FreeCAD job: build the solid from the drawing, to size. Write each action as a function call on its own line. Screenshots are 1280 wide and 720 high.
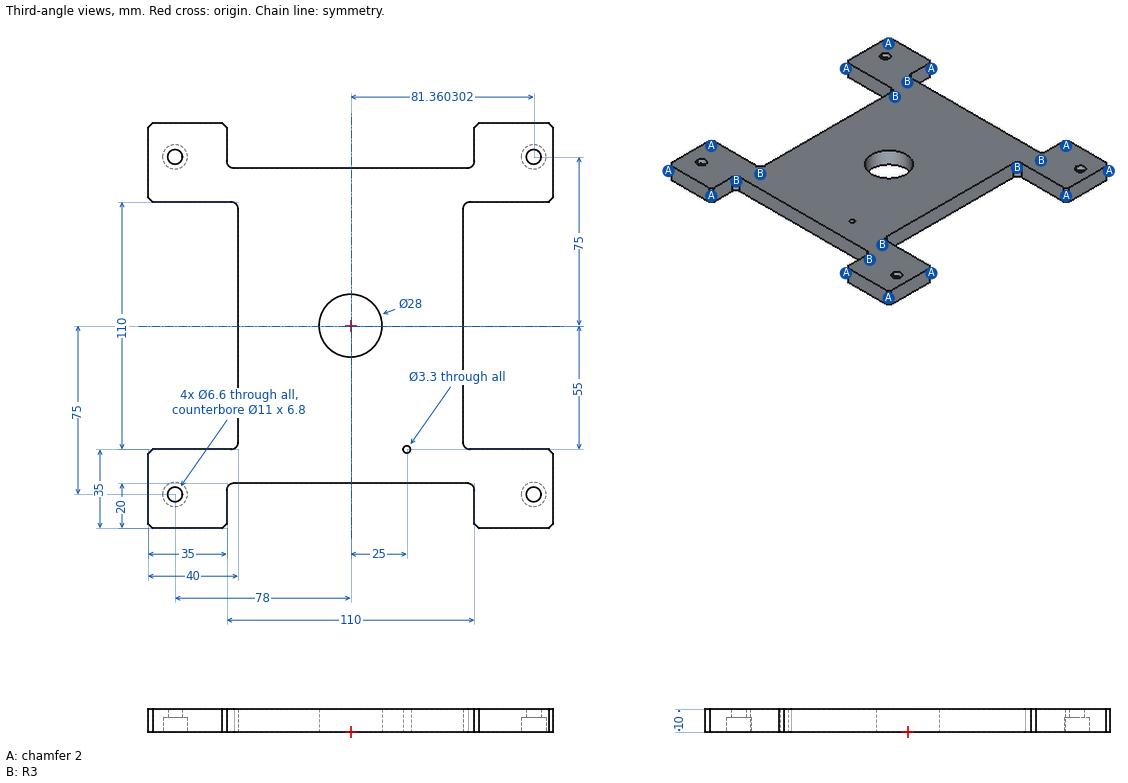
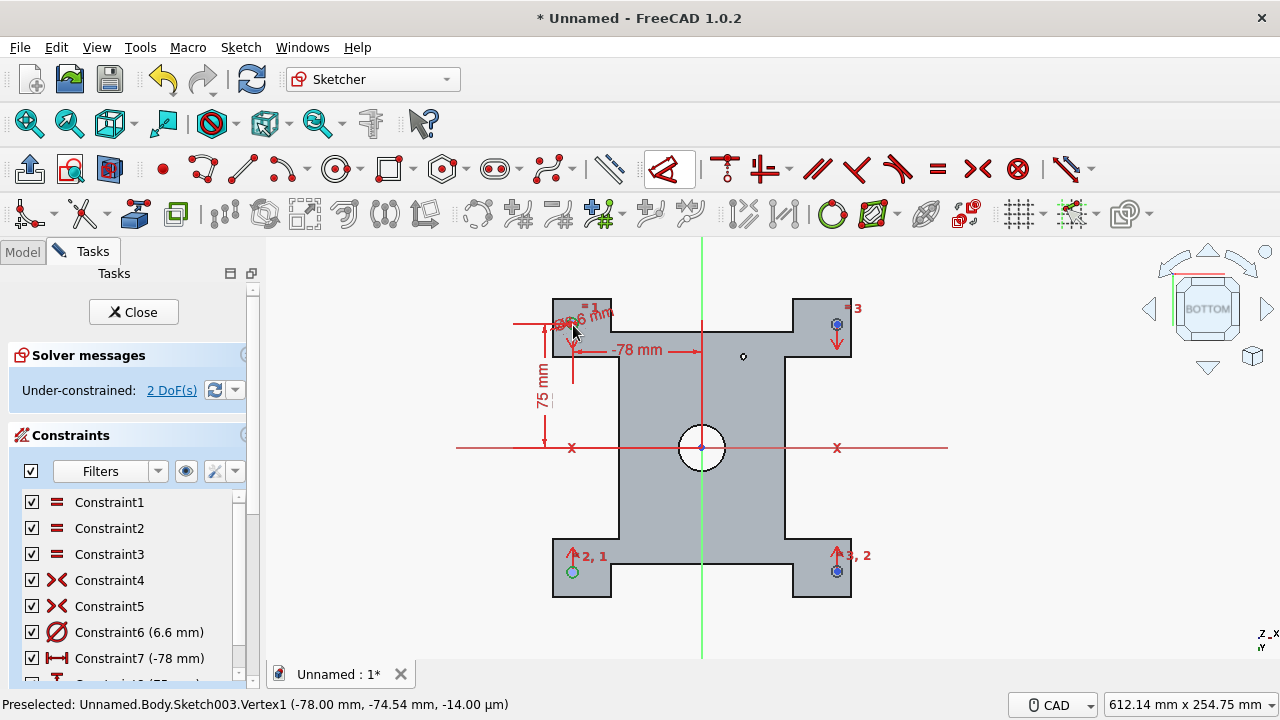
click(837, 571)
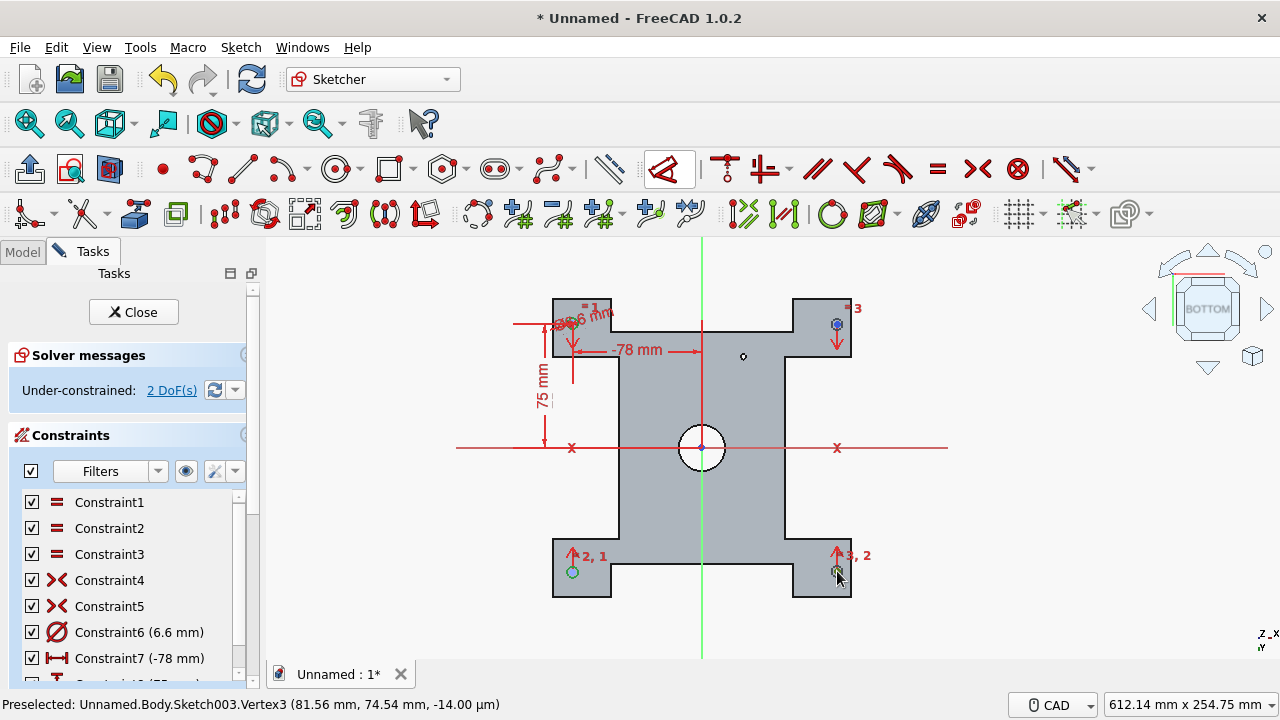
key(i)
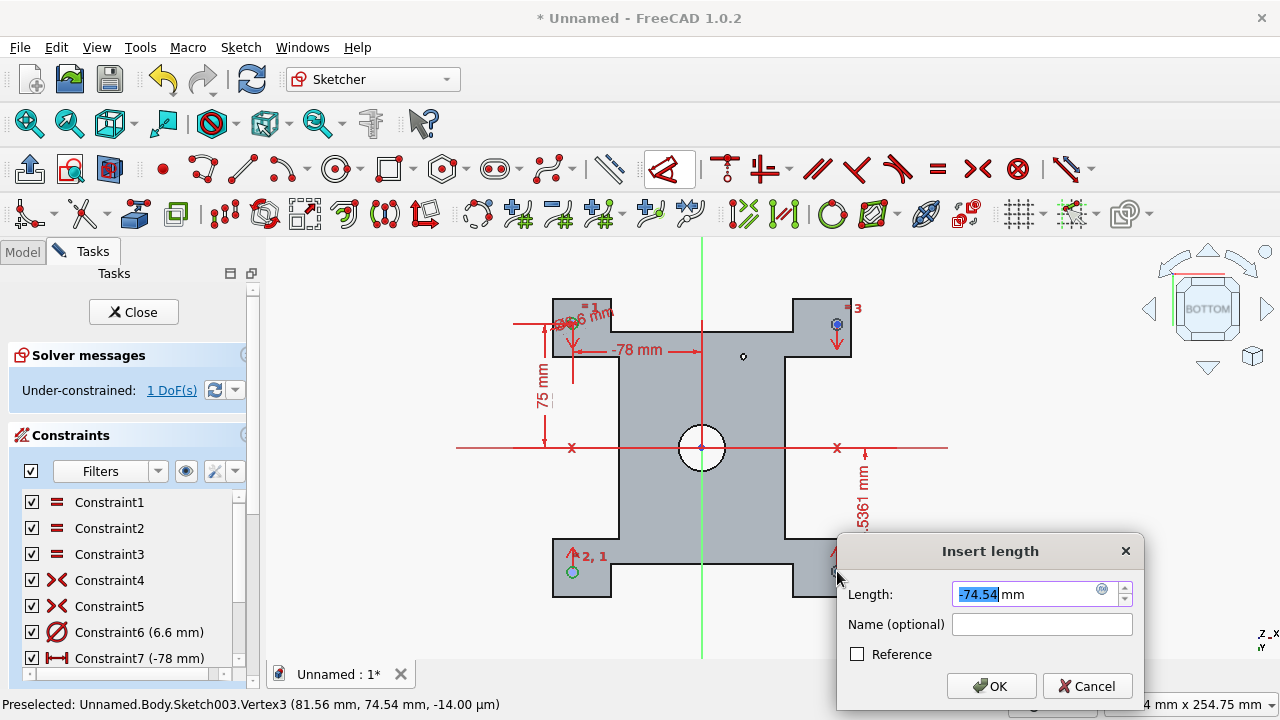
text(-75)
key(Return)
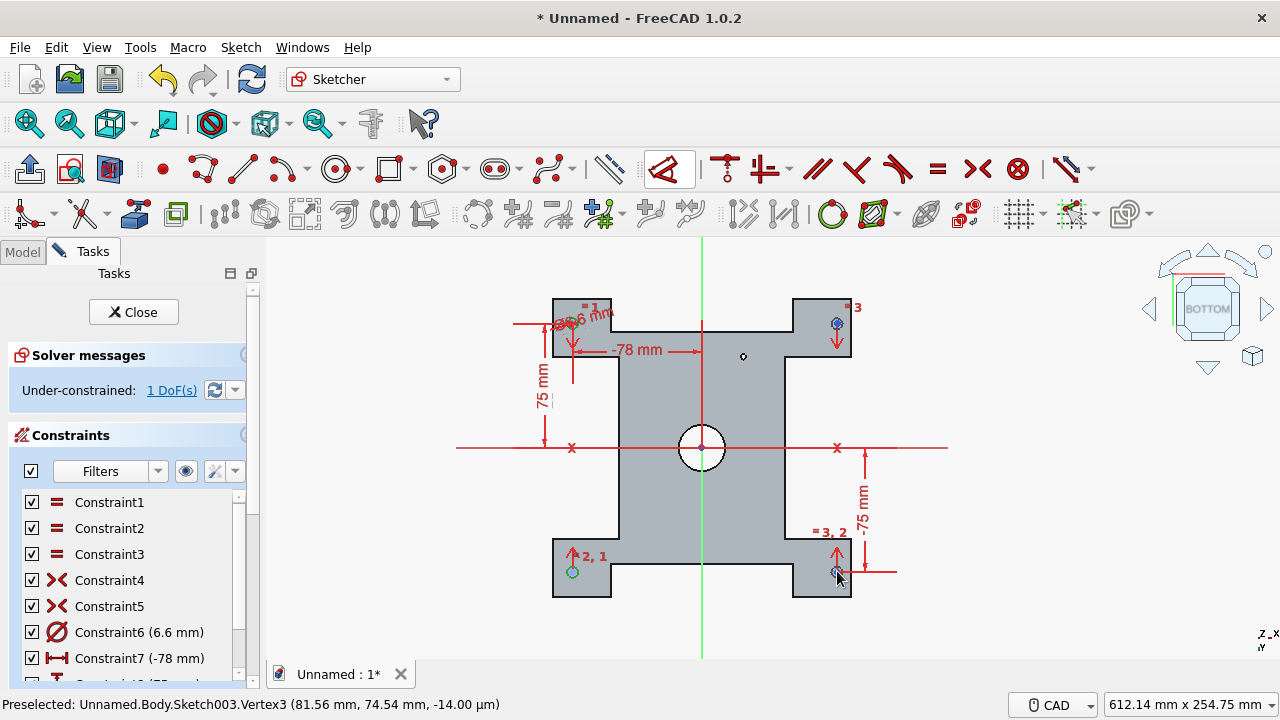
click(837, 572)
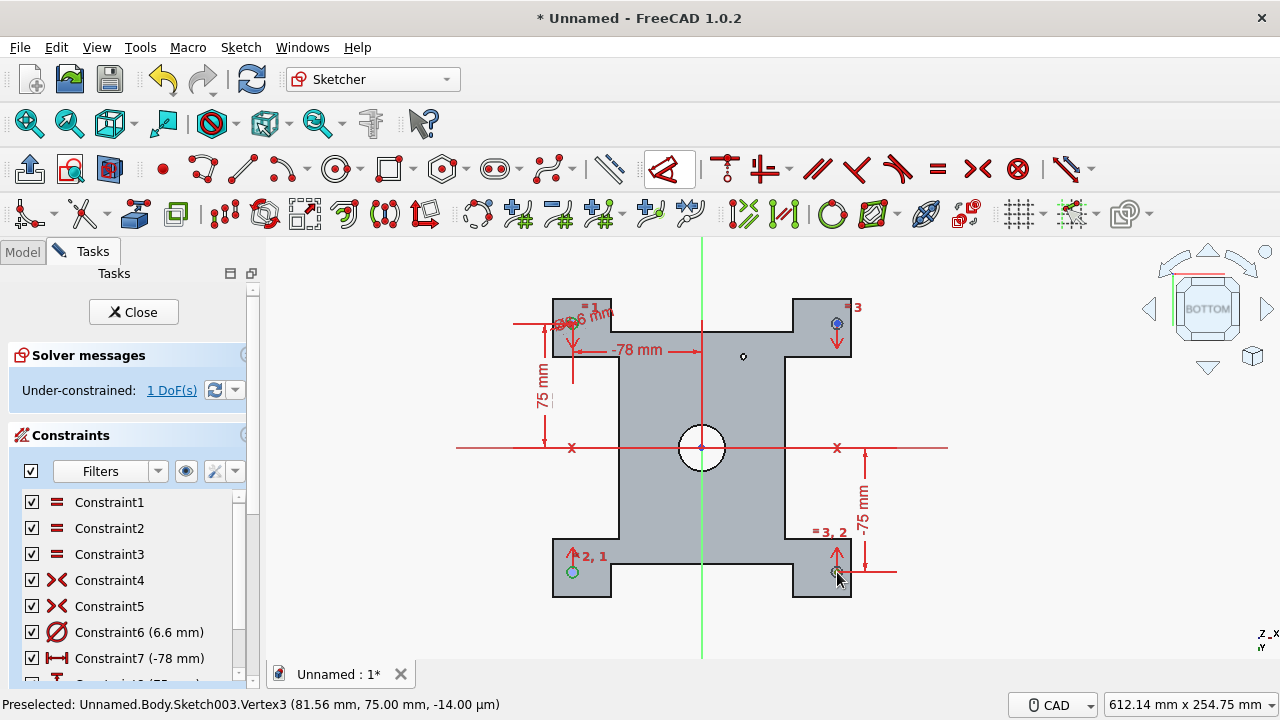
key(l)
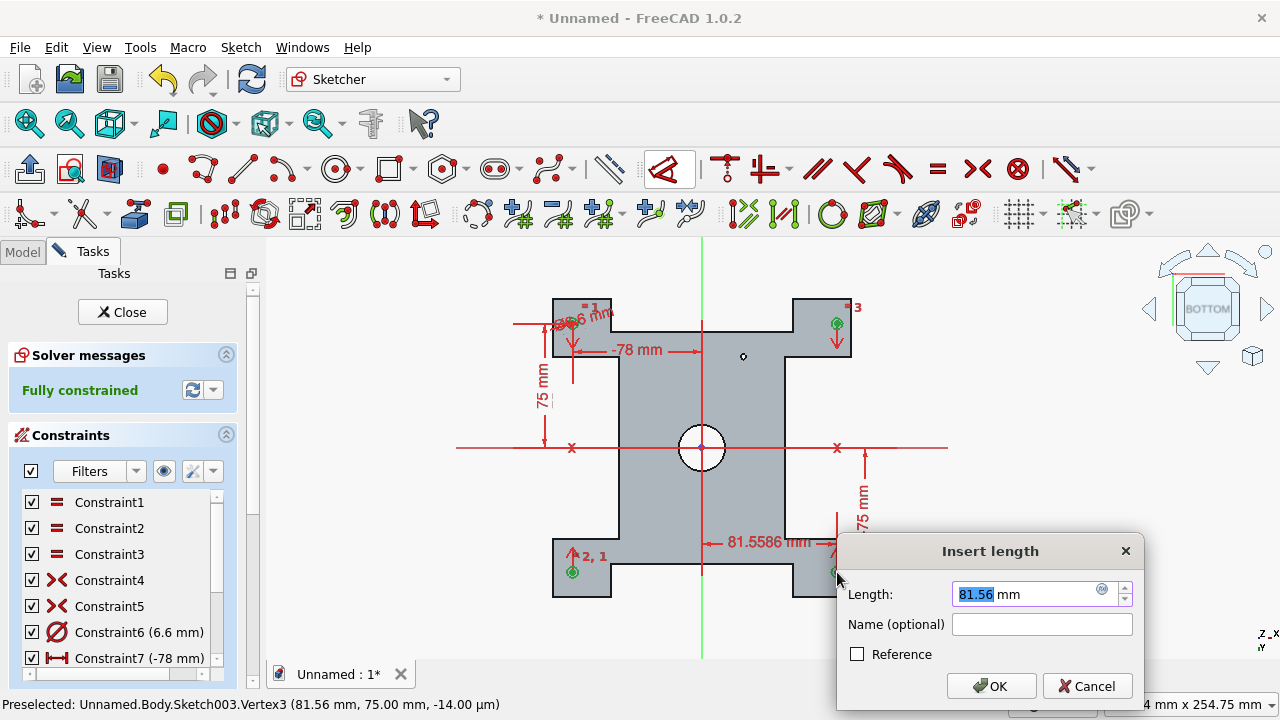
text(81.360302)
key(Return)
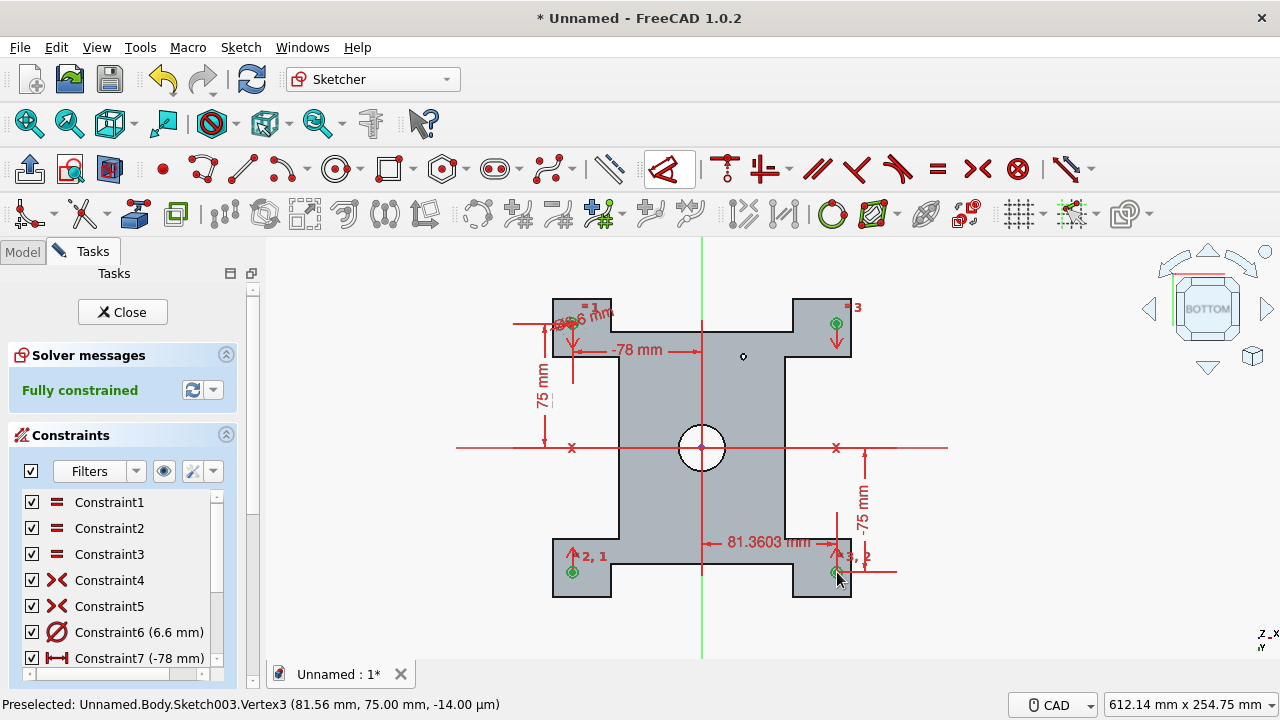
click(123, 312)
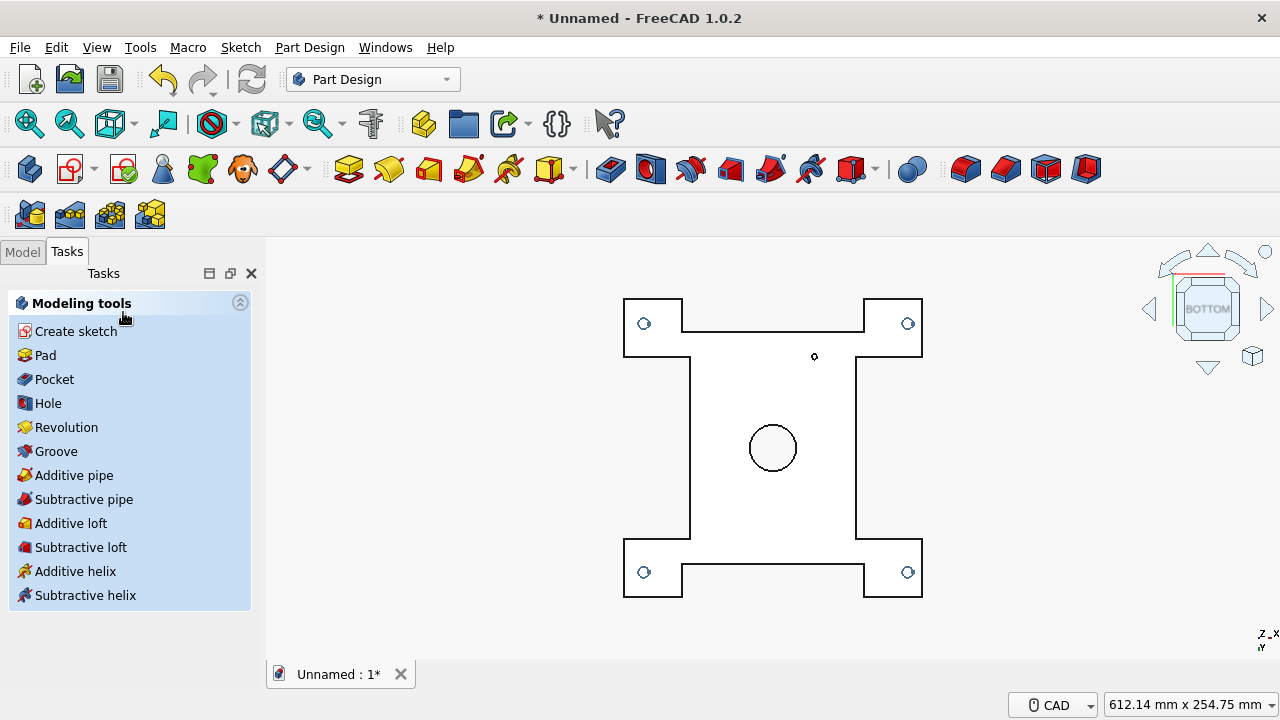
click(652, 170)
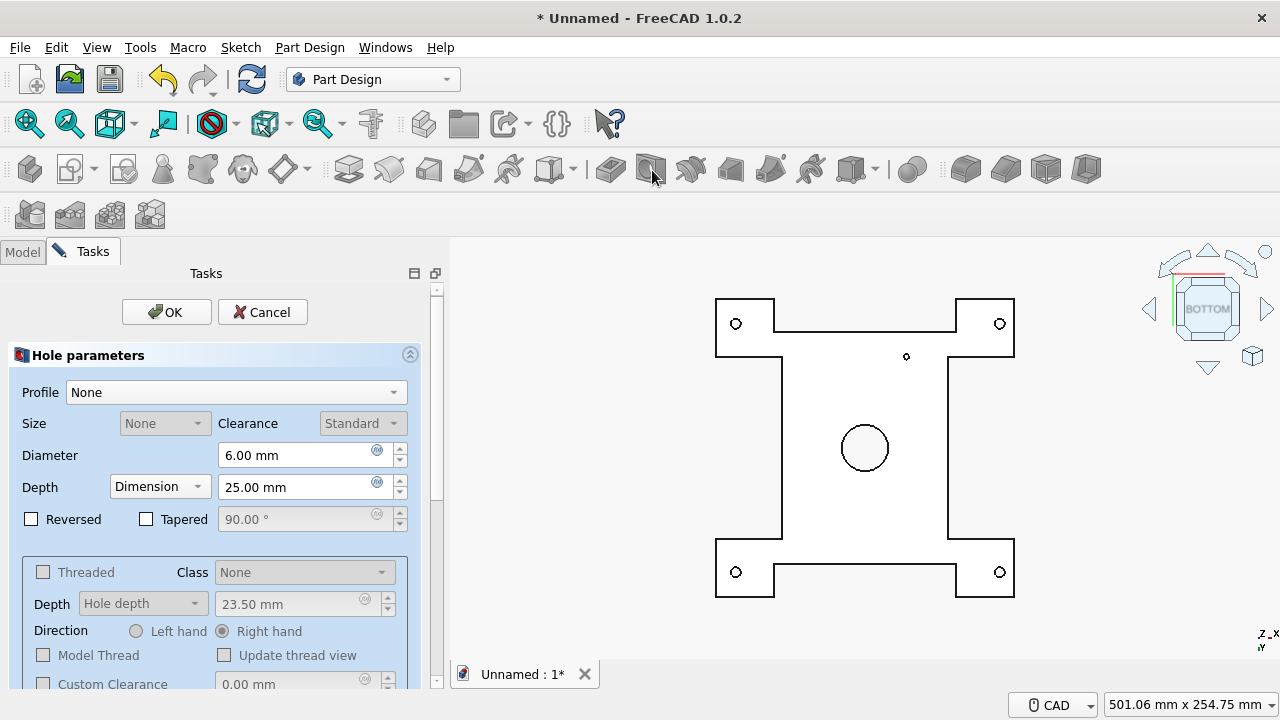
triple_click(305, 455)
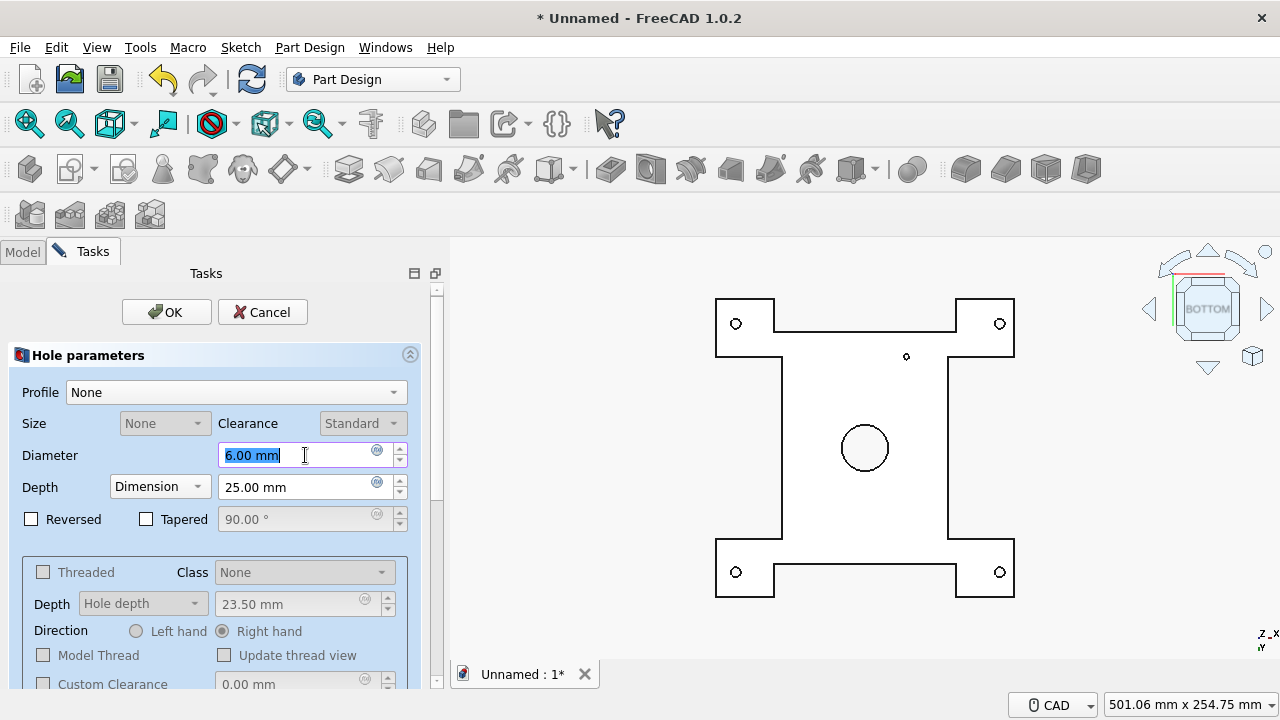
text(6.6)
key(Tab)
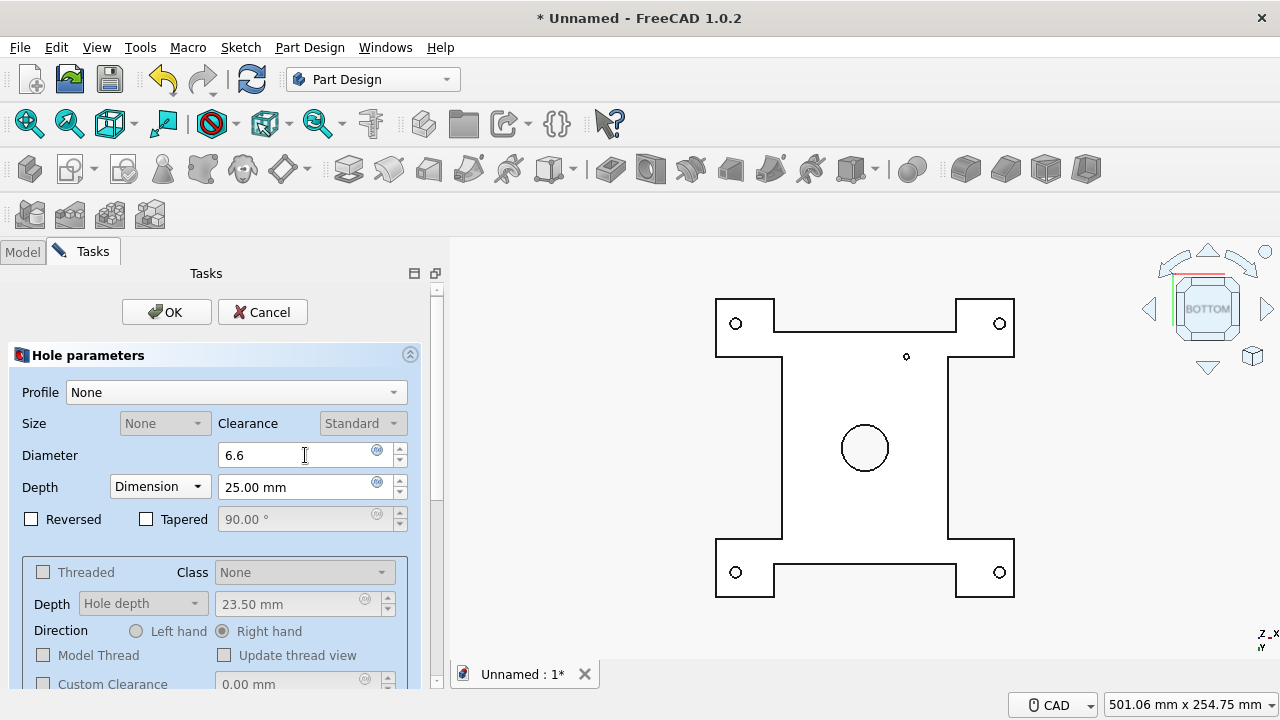
click(161, 486)